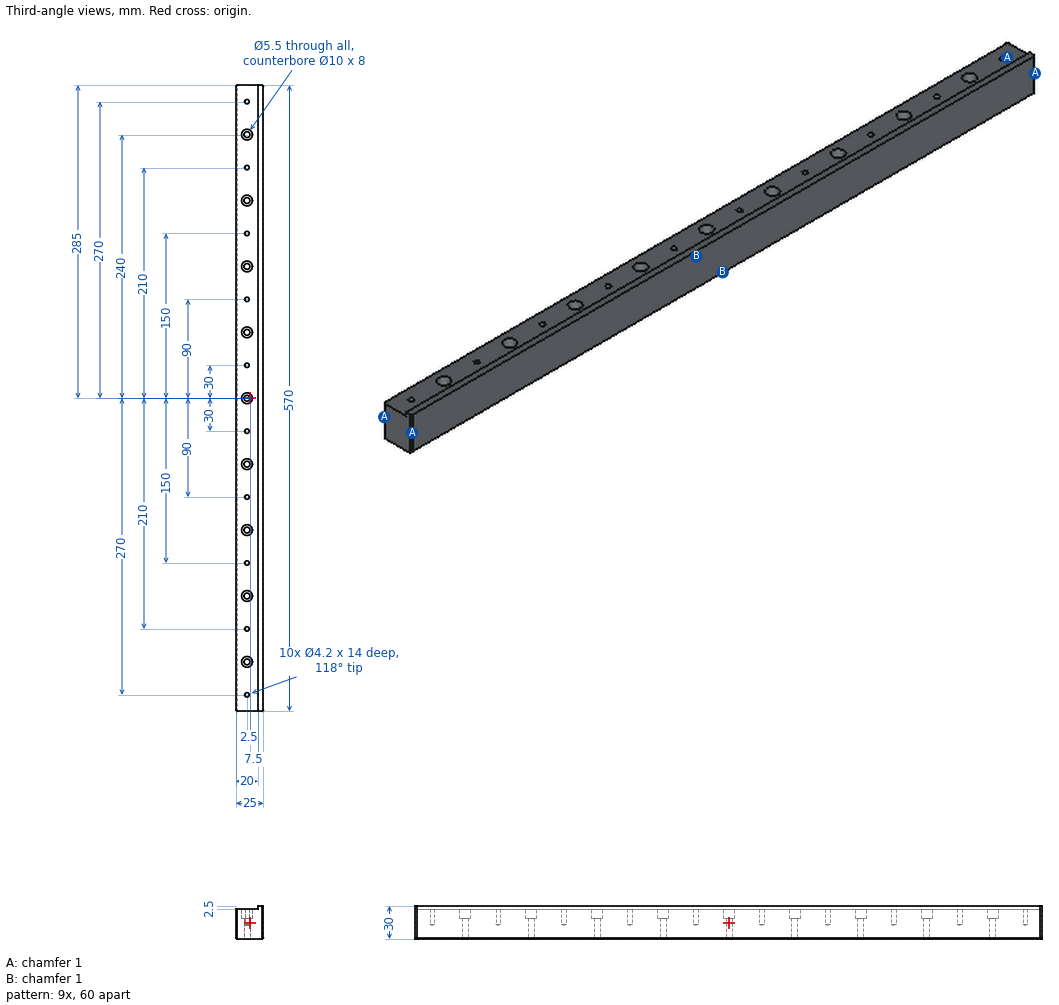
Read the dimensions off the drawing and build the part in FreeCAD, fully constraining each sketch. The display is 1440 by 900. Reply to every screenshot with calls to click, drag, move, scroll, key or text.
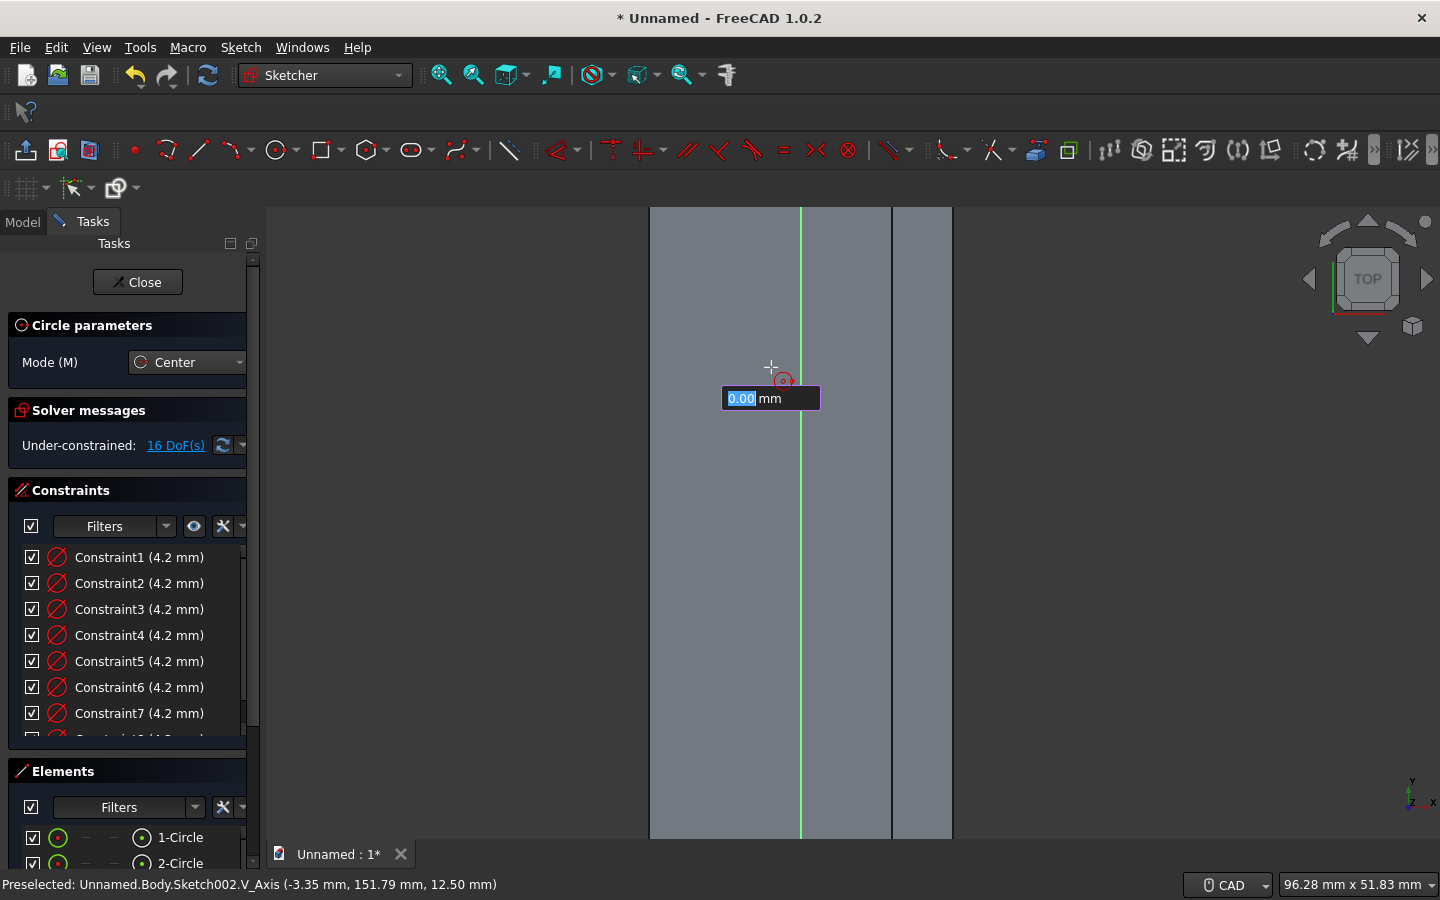
scroll(785, 367, down, 14)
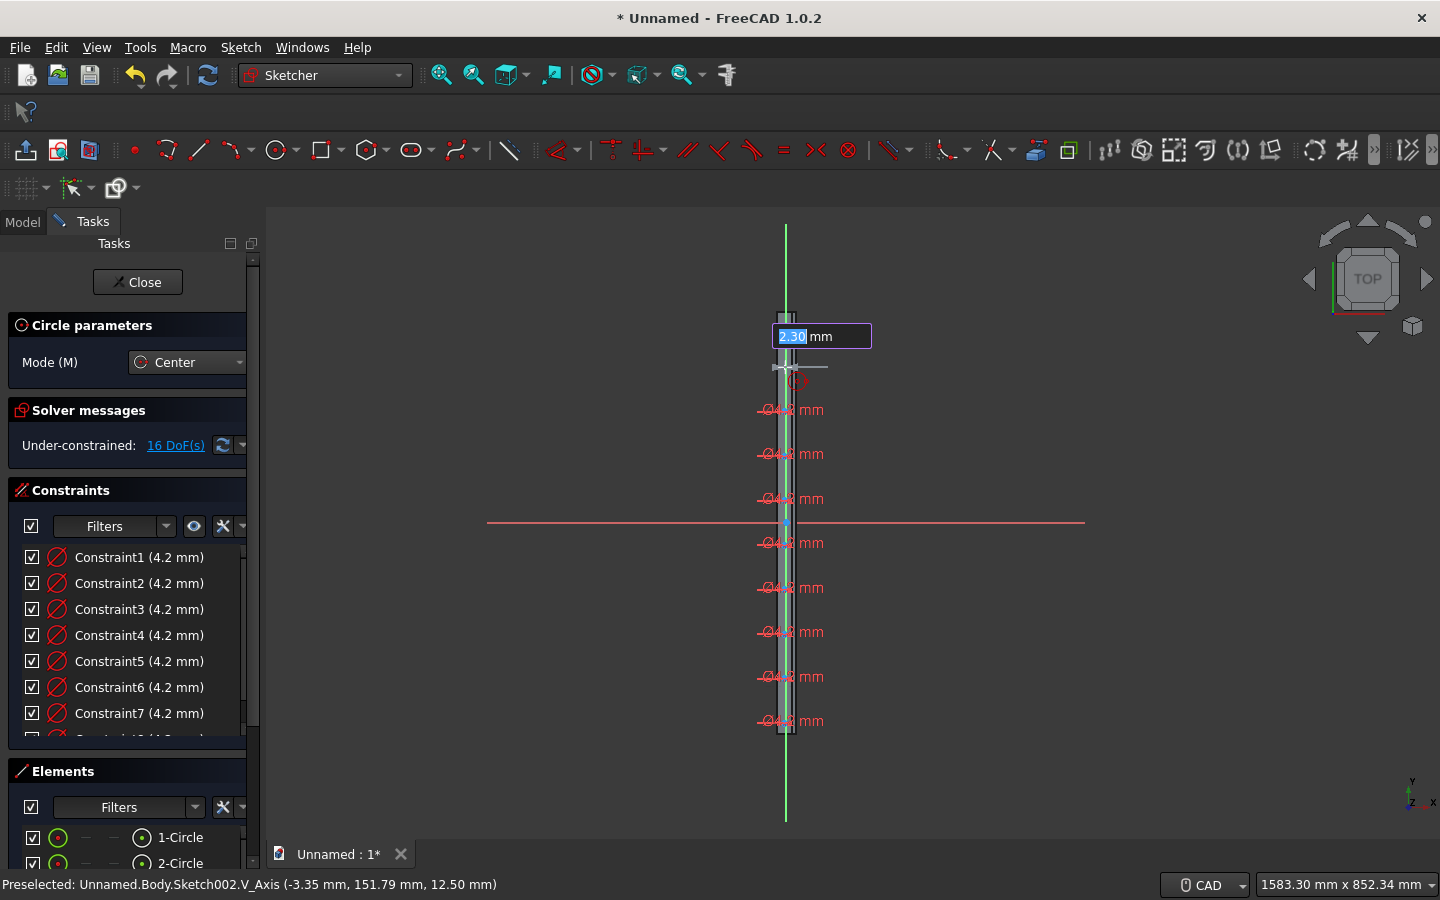
scroll(783, 366, up, 9)
move(783, 366)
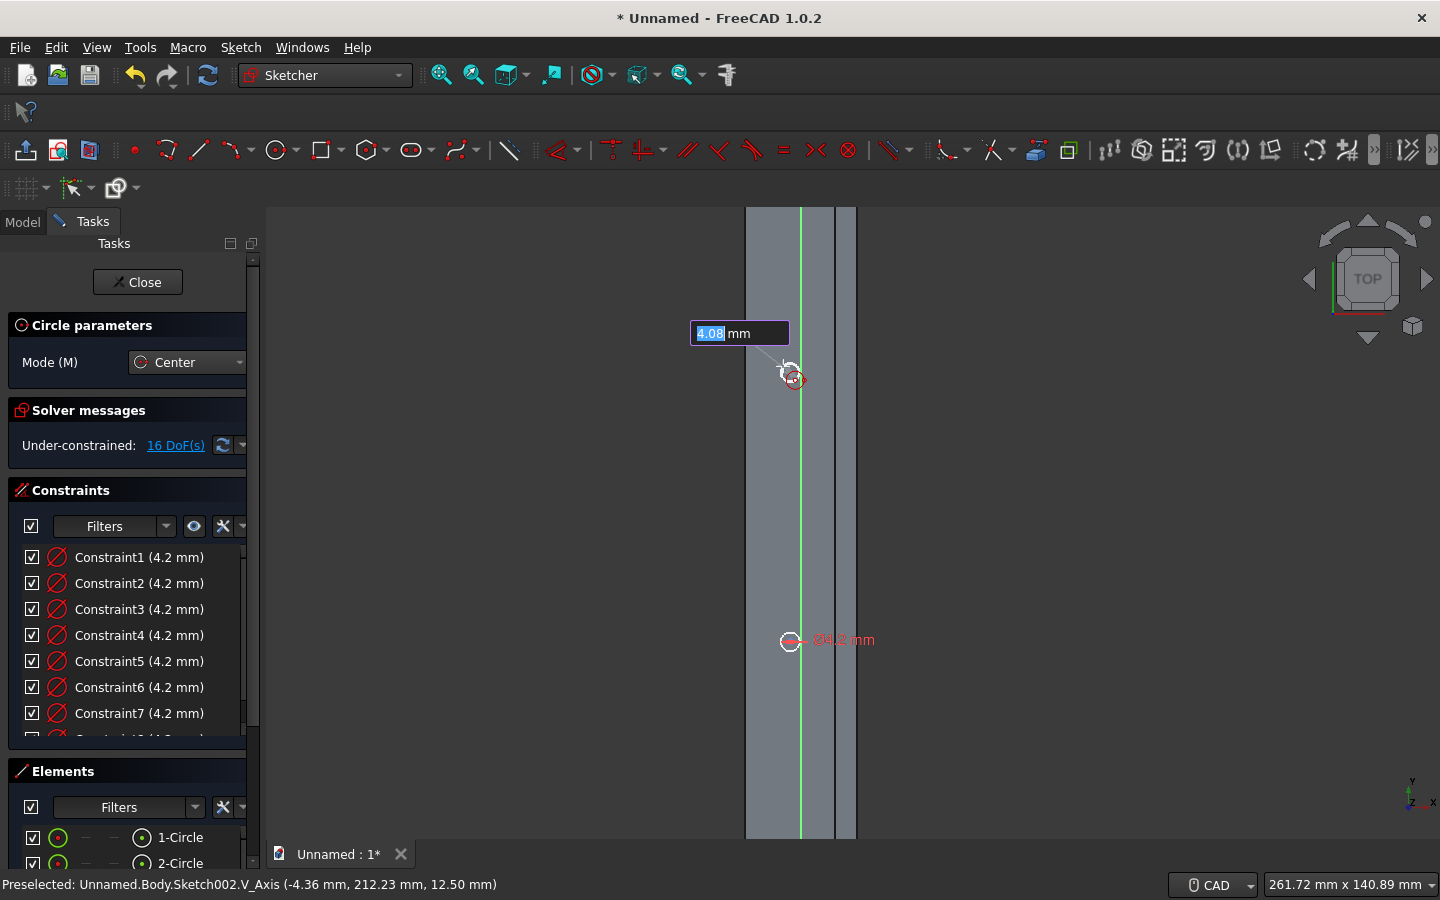
text(4.2)
key(Return)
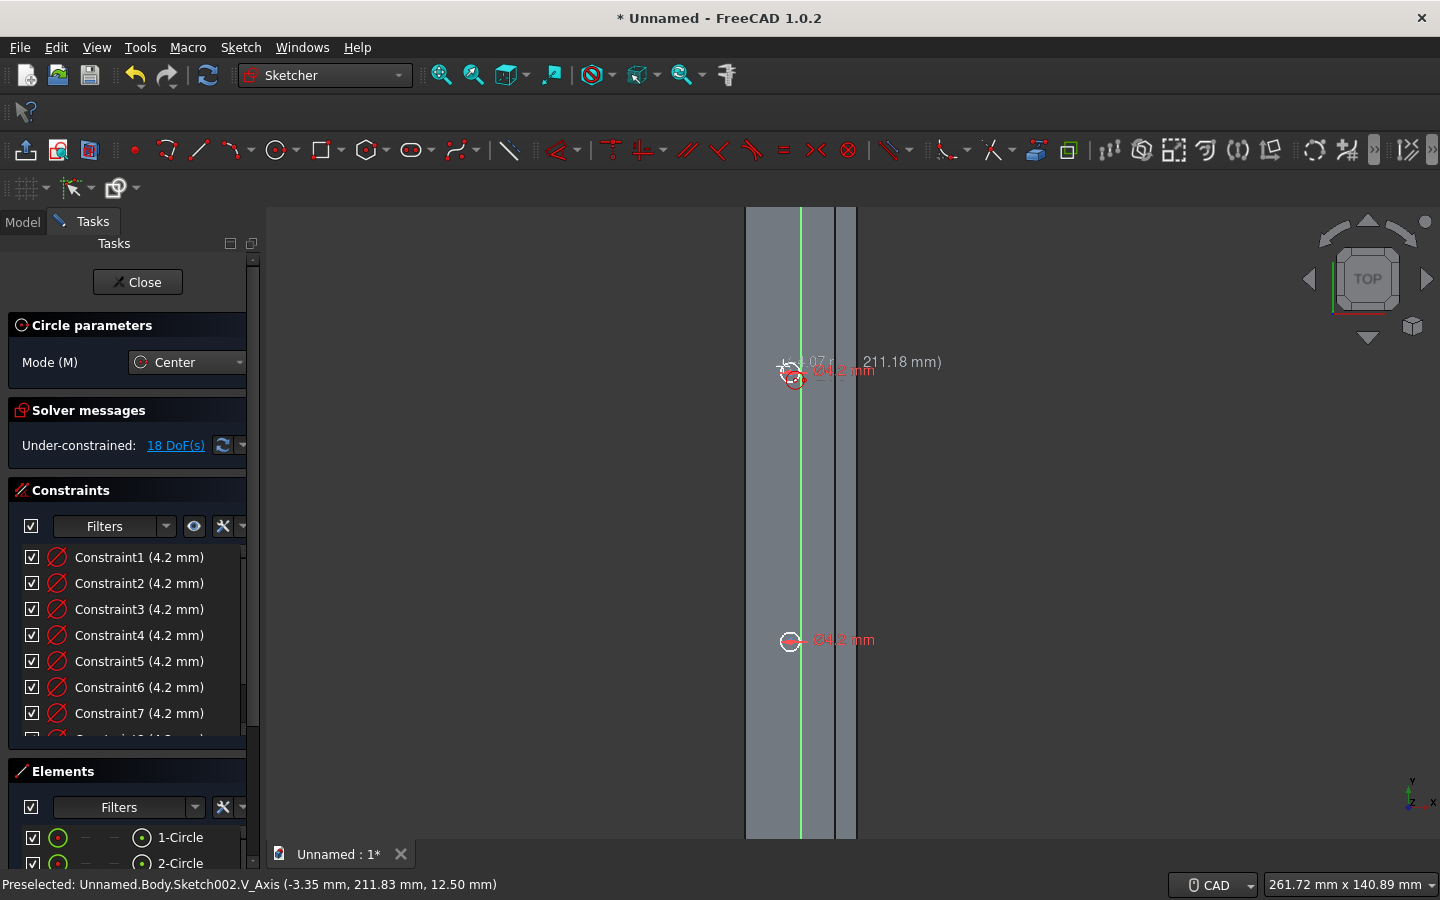
scroll(783, 366, down, 9)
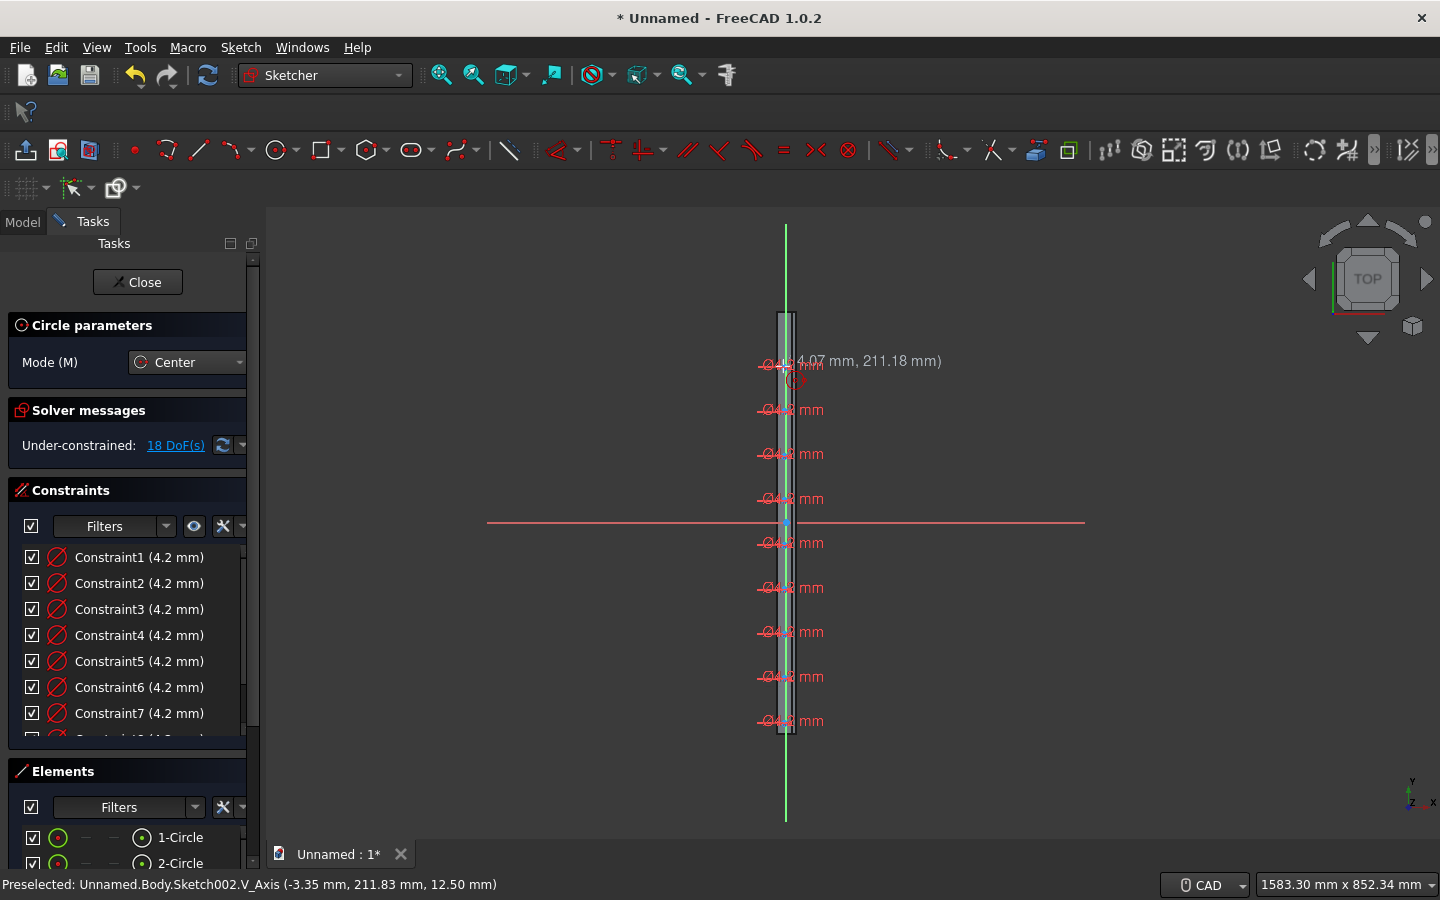
scroll(785, 323, up, 14)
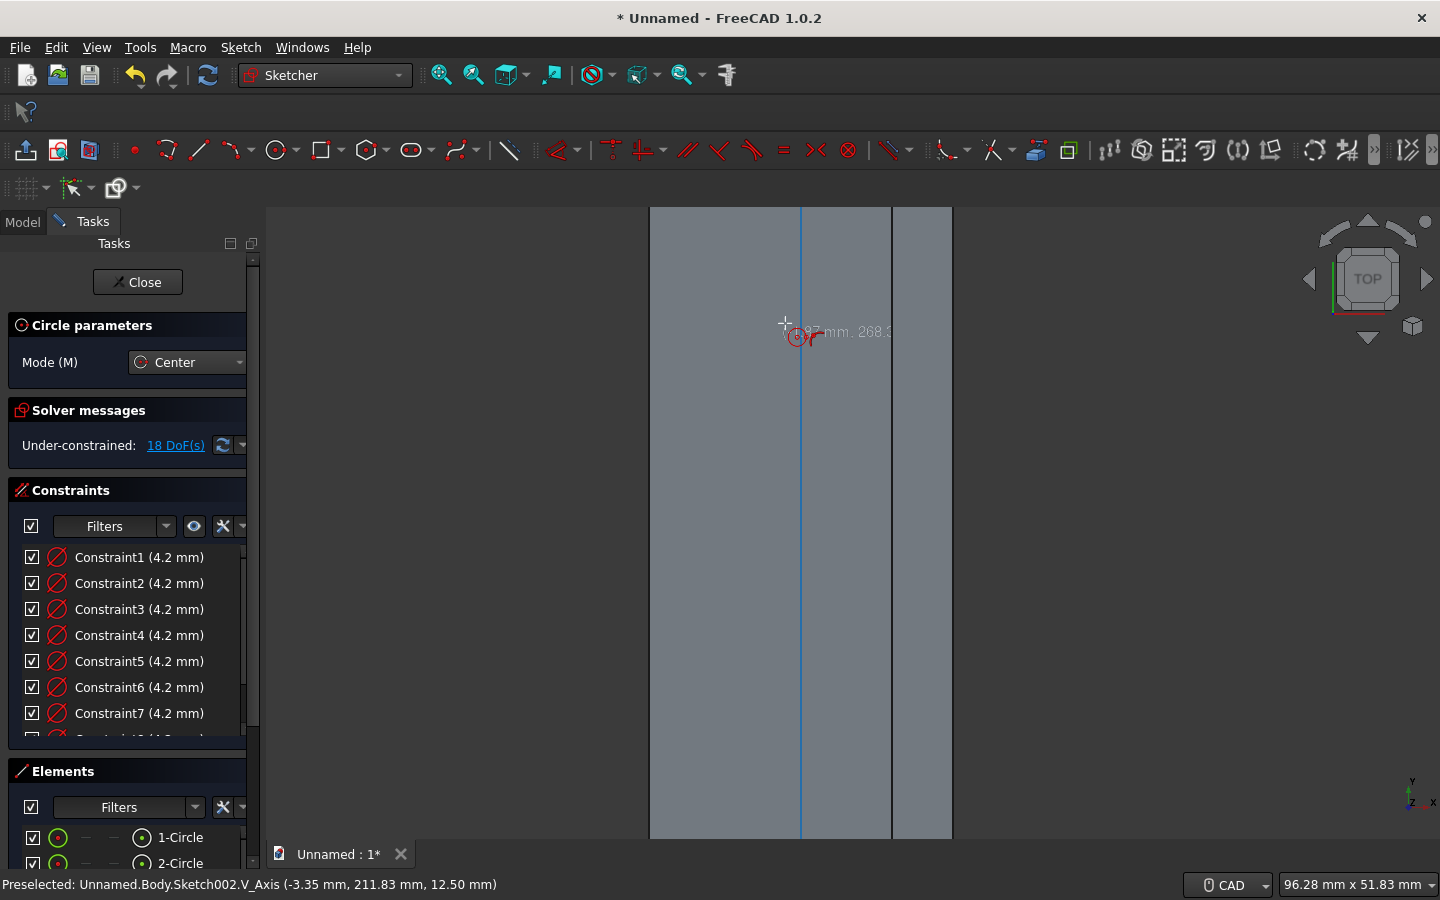
click(771, 316)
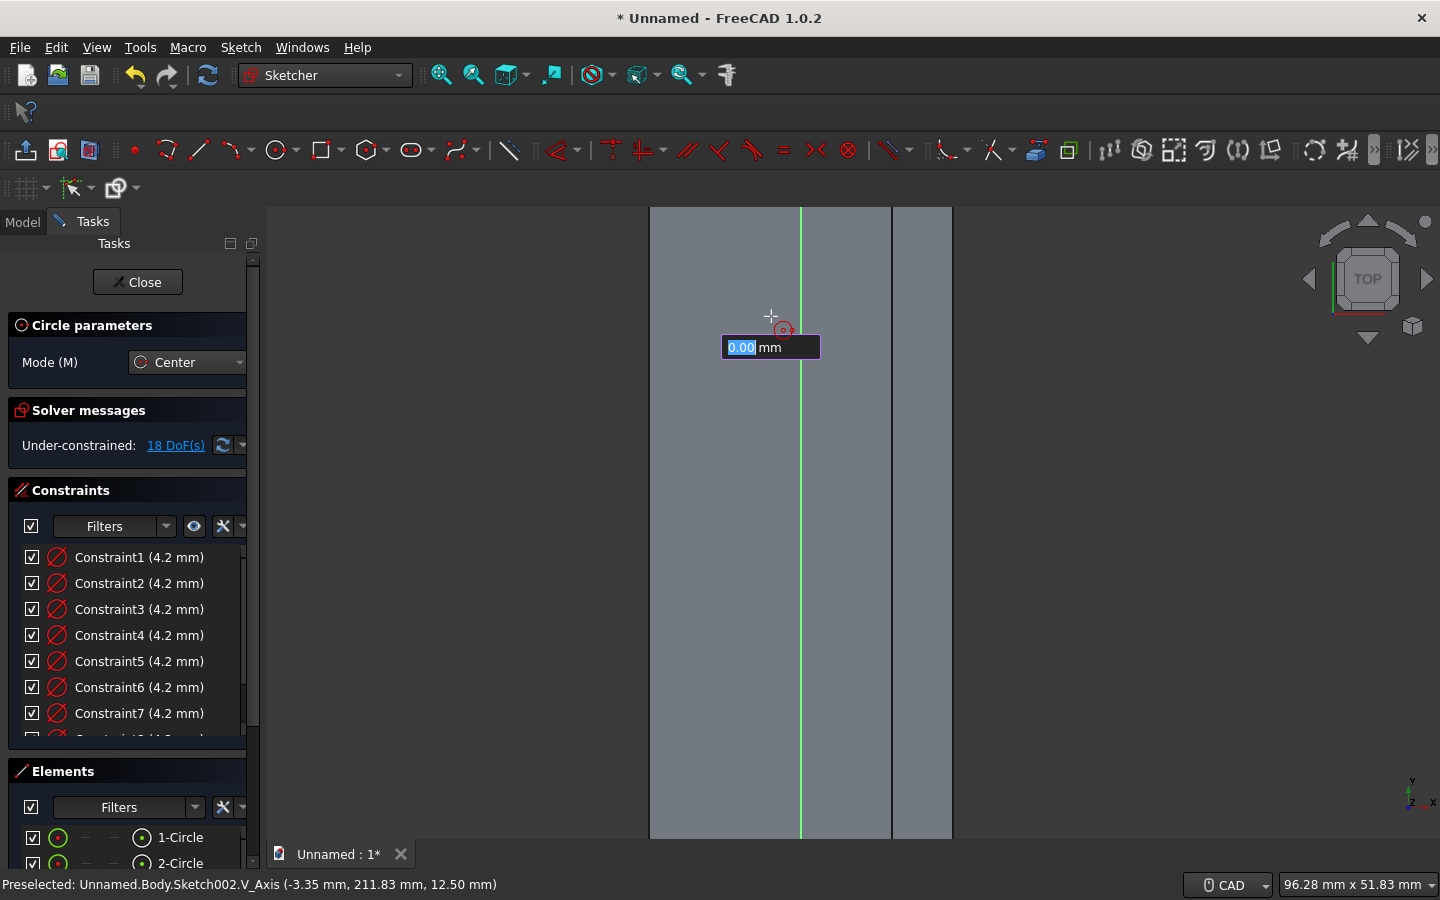
scroll(785, 323, down, 14)